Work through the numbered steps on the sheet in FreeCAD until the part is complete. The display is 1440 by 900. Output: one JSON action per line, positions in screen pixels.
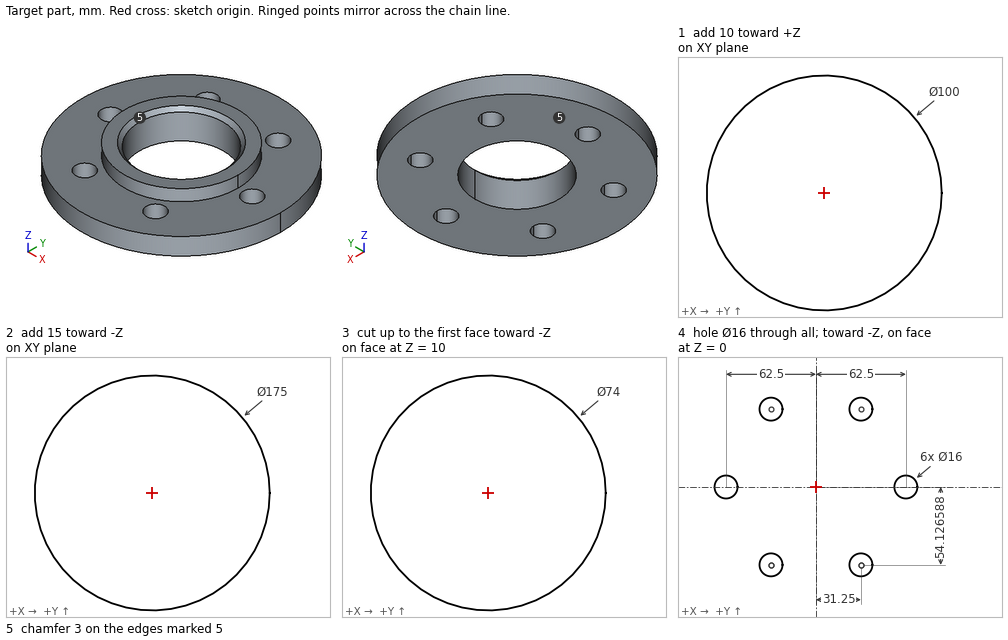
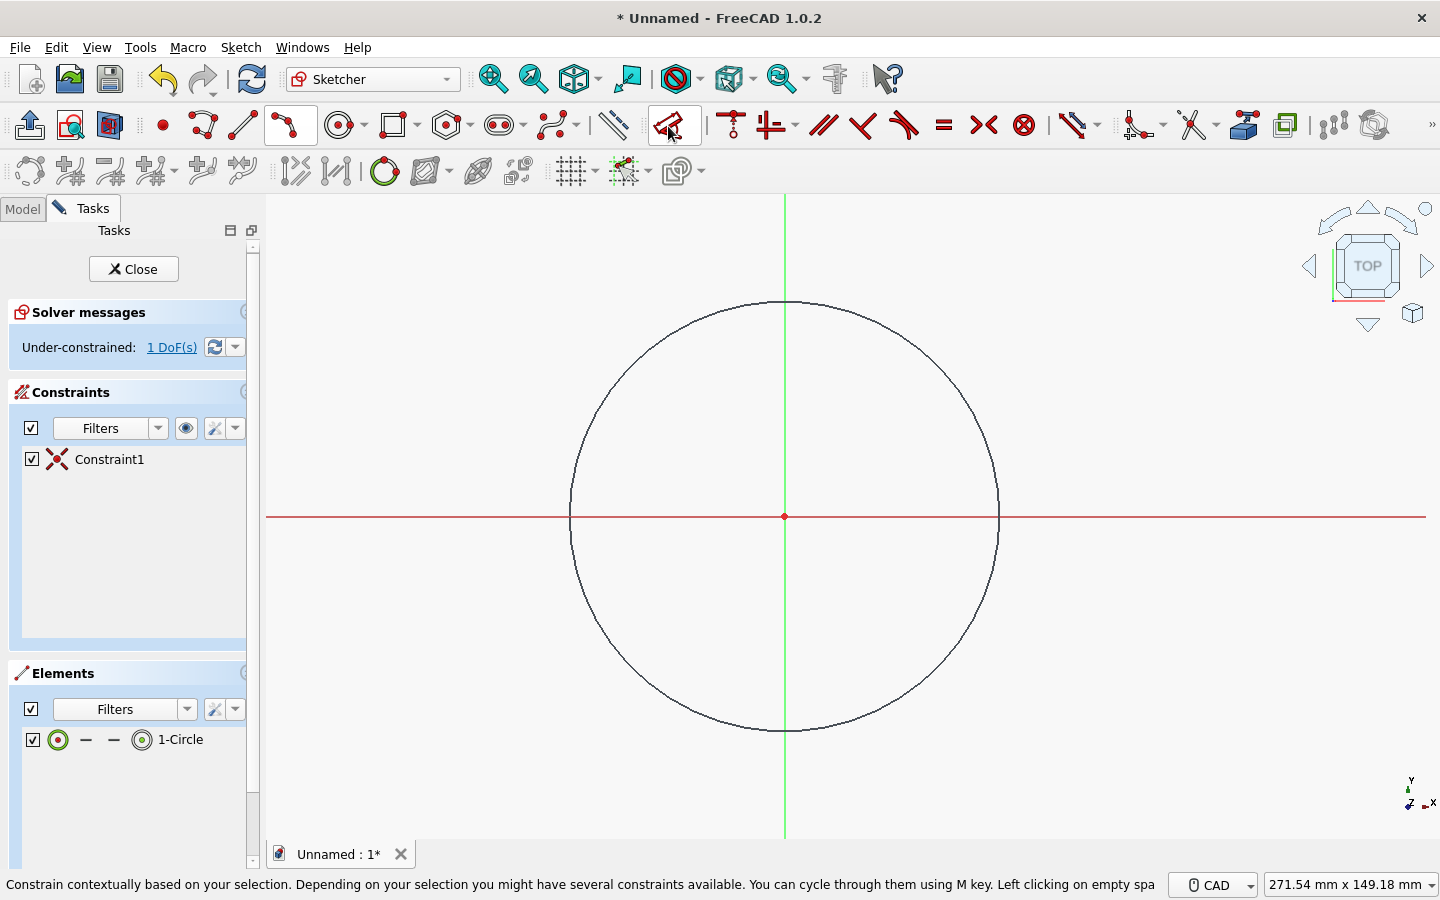
{"action": "left_click", "coordinate": [936, 364]}
{"action": "left_click", "coordinate": [959, 341]}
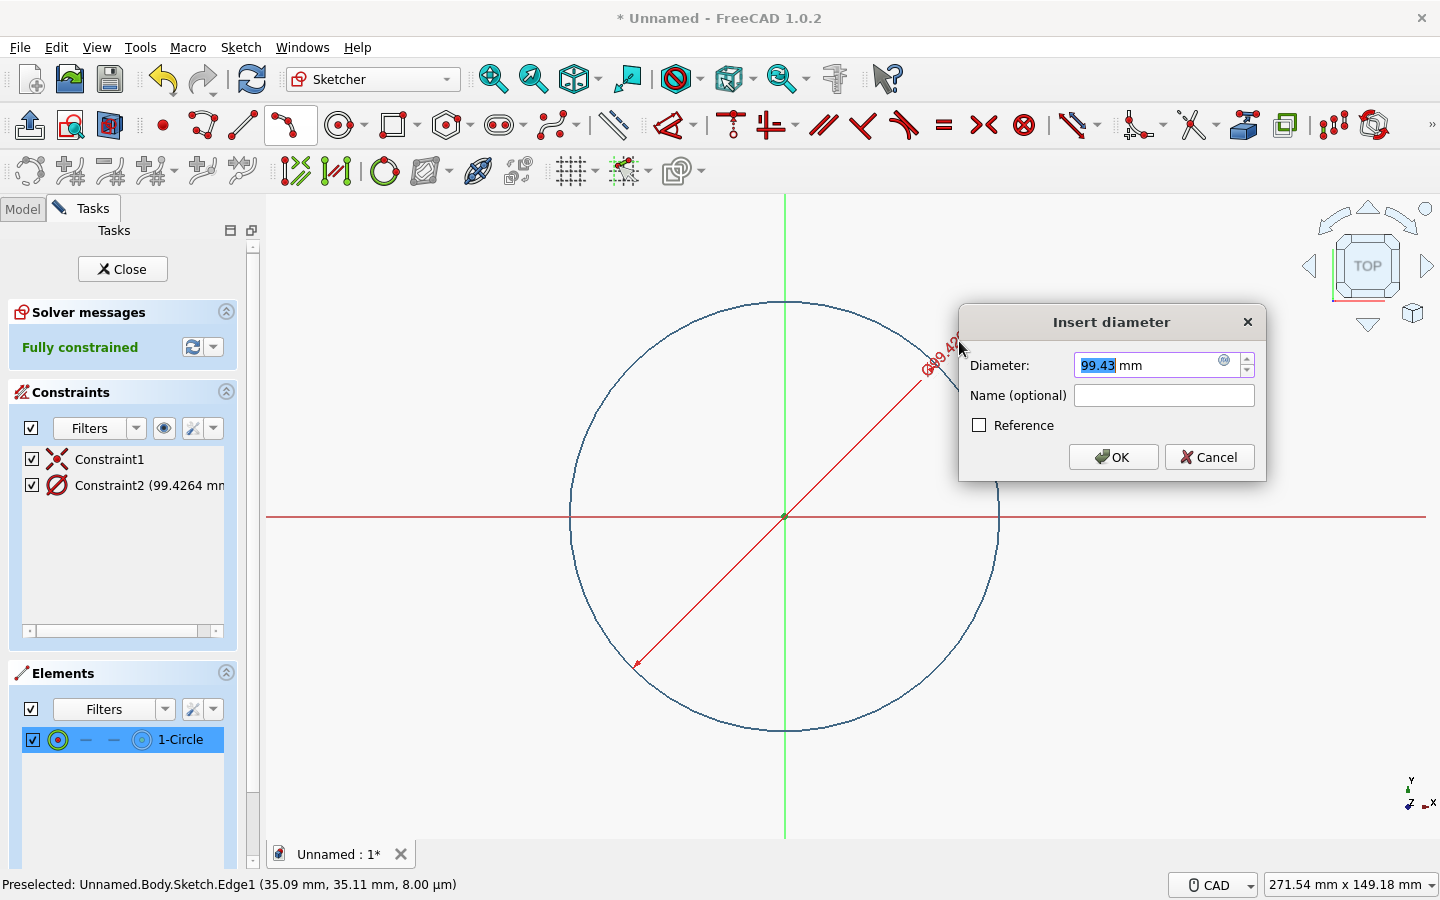
{"action": "type", "text": "100"}
{"action": "key", "text": "Return"}
{"action": "key", "text": "Escape"}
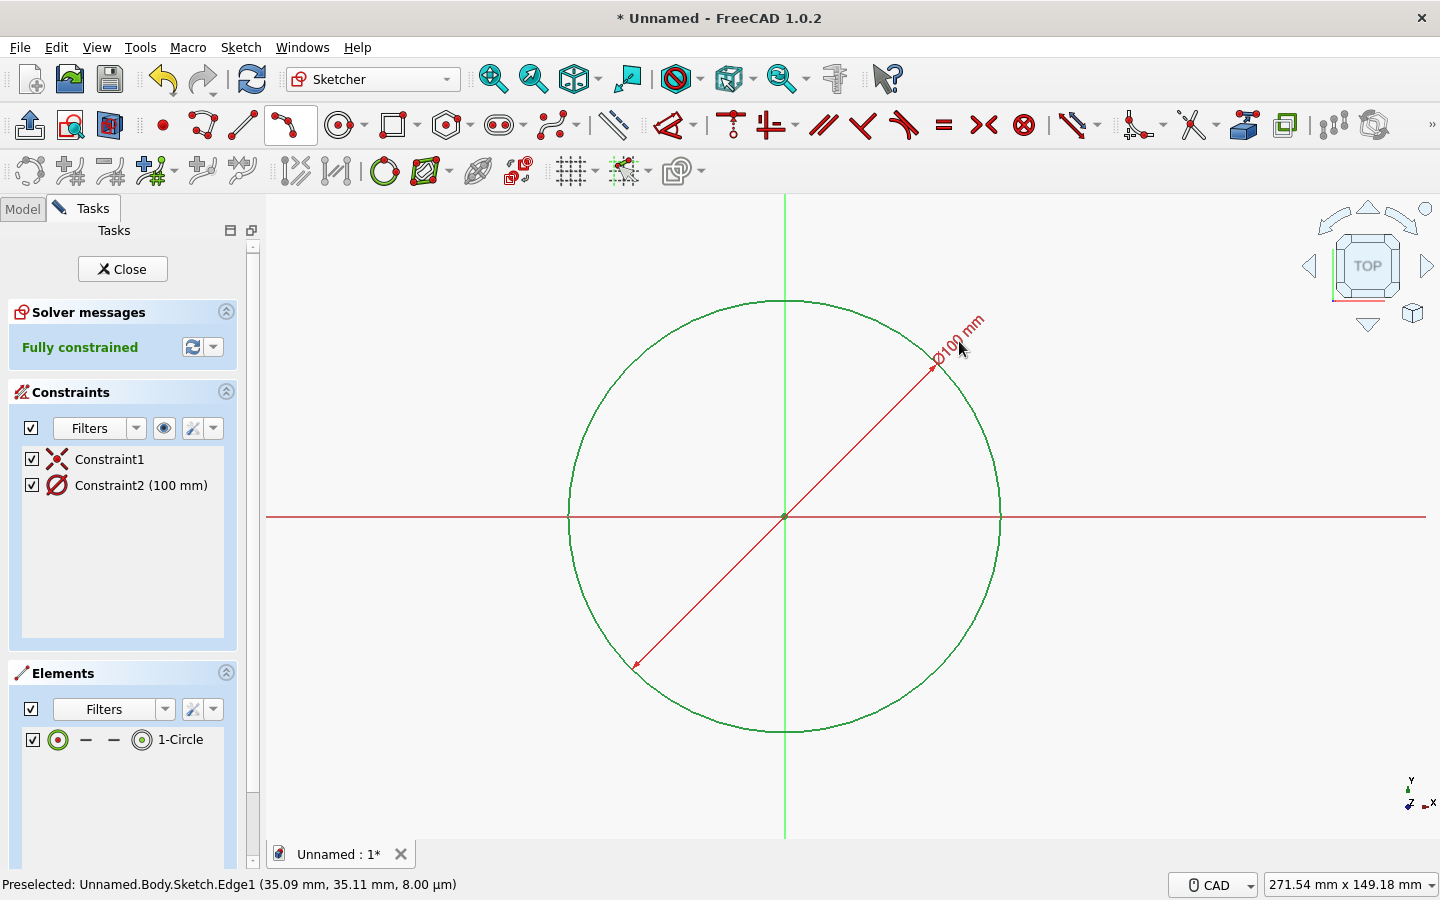
{"action": "left_click", "coordinate": [123, 269]}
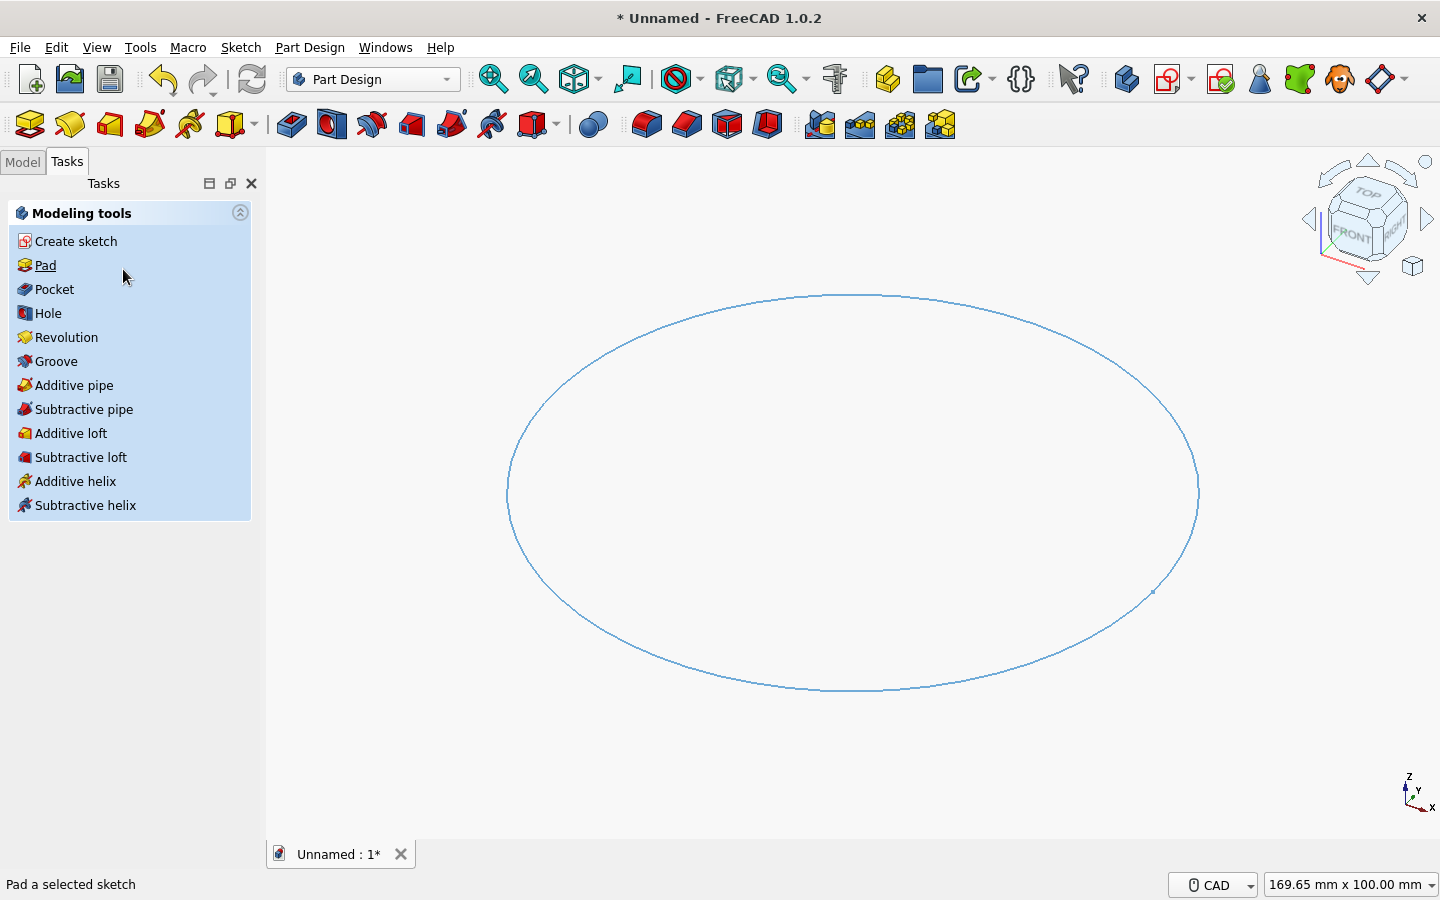
{"action": "left_click", "coordinate": [30, 124]}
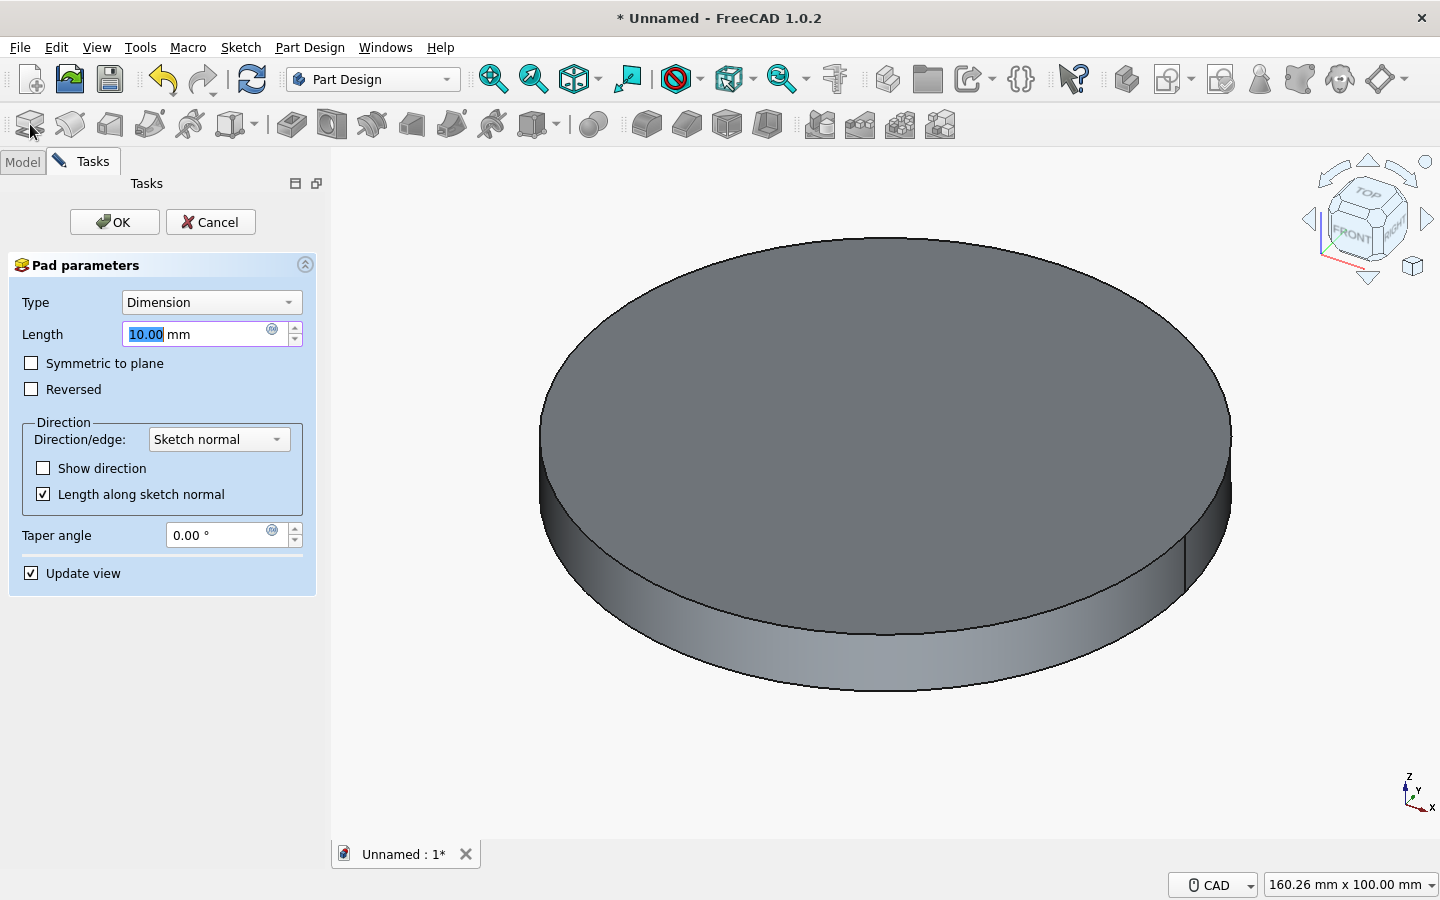
{"action": "type", "text": "10"}
{"action": "key", "text": "Tab"}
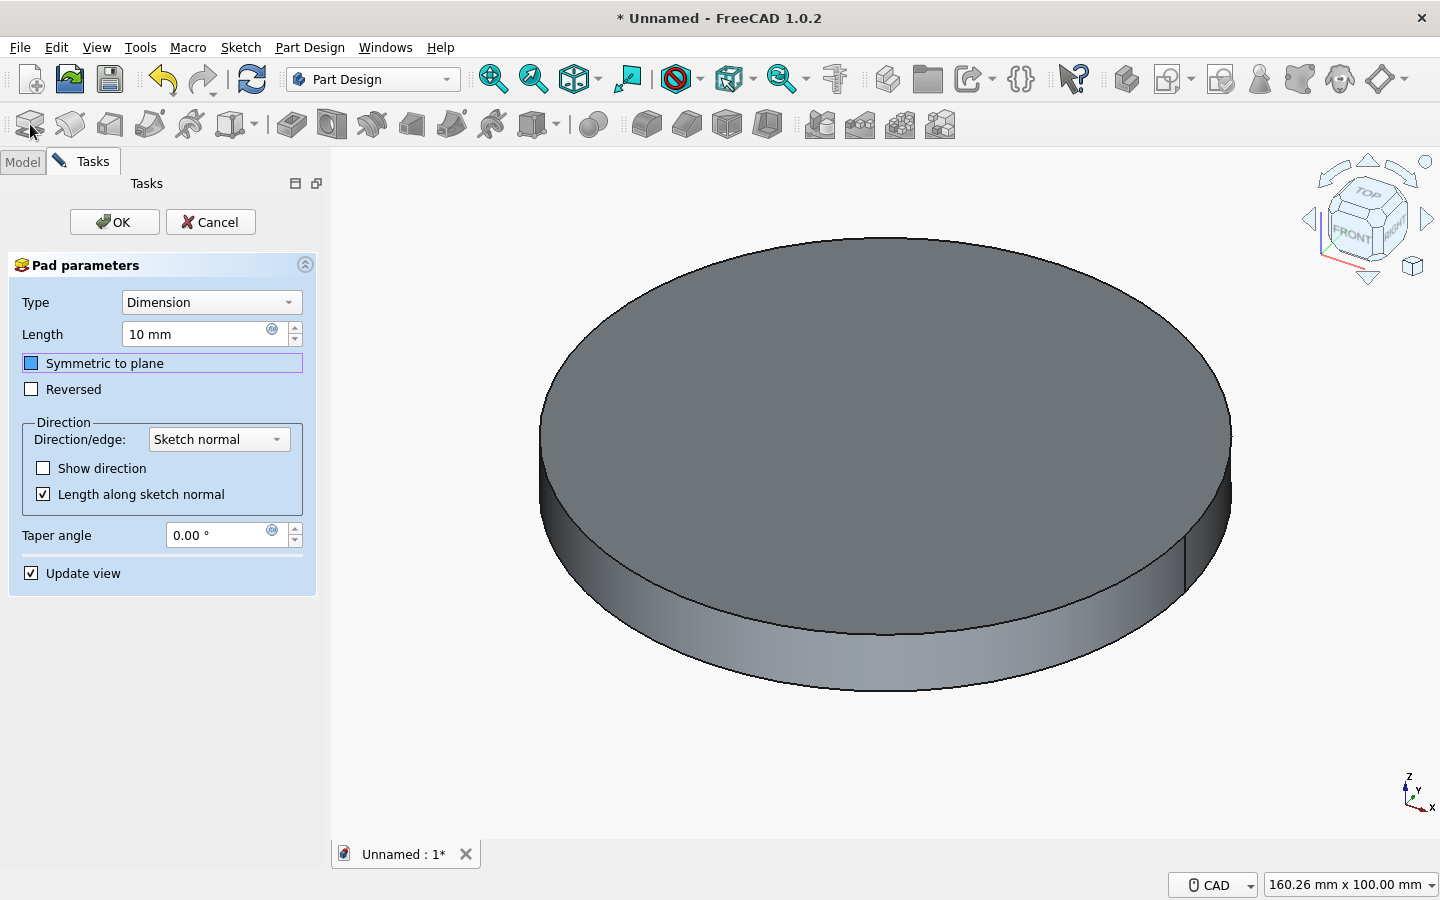
{"action": "left_click", "coordinate": [115, 222]}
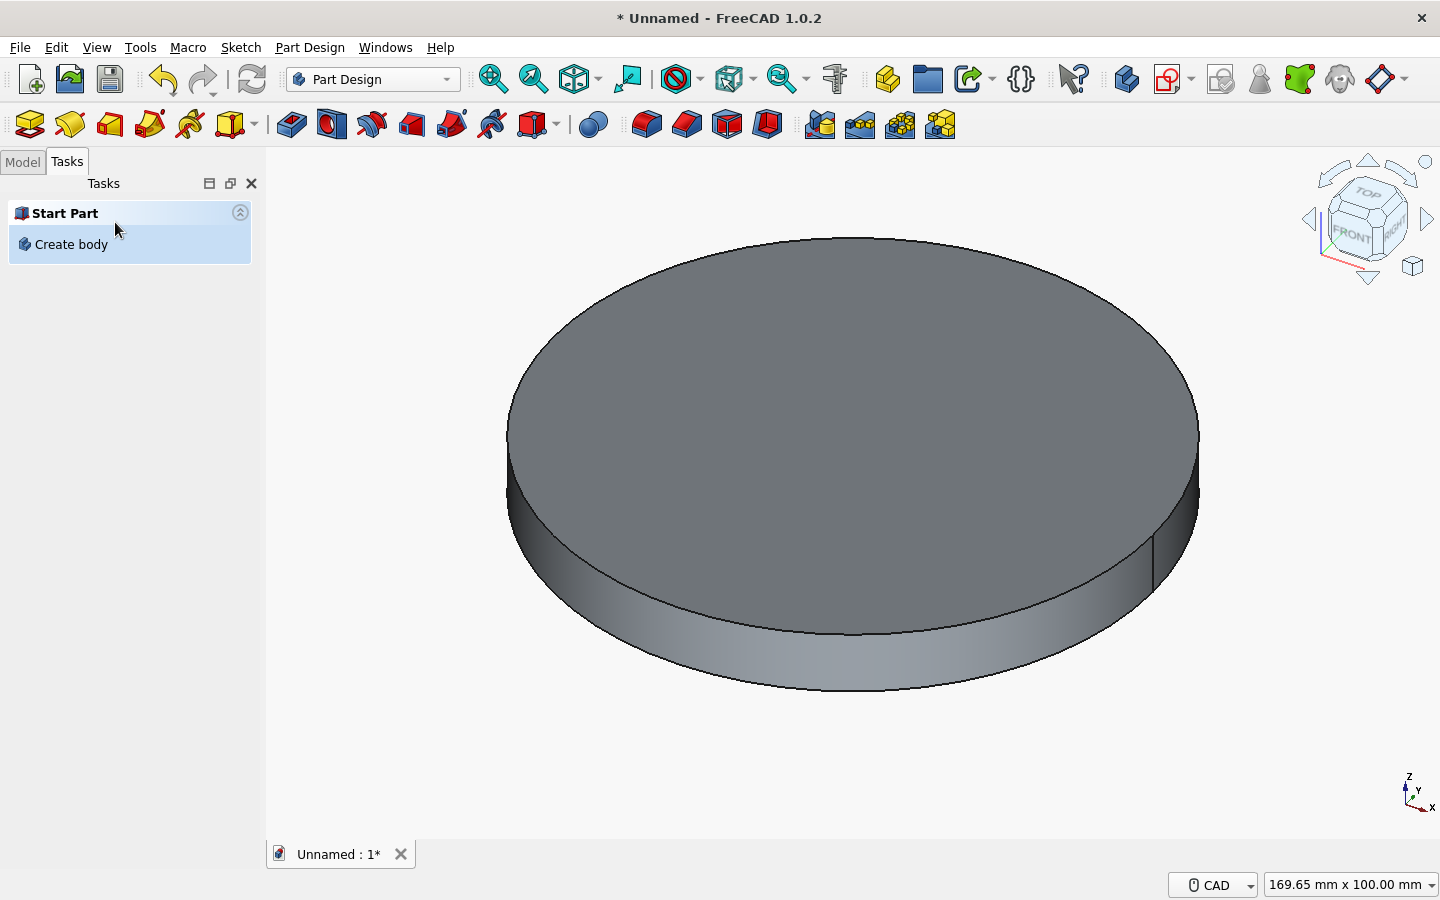
{"action": "left_click", "coordinate": [1168, 80]}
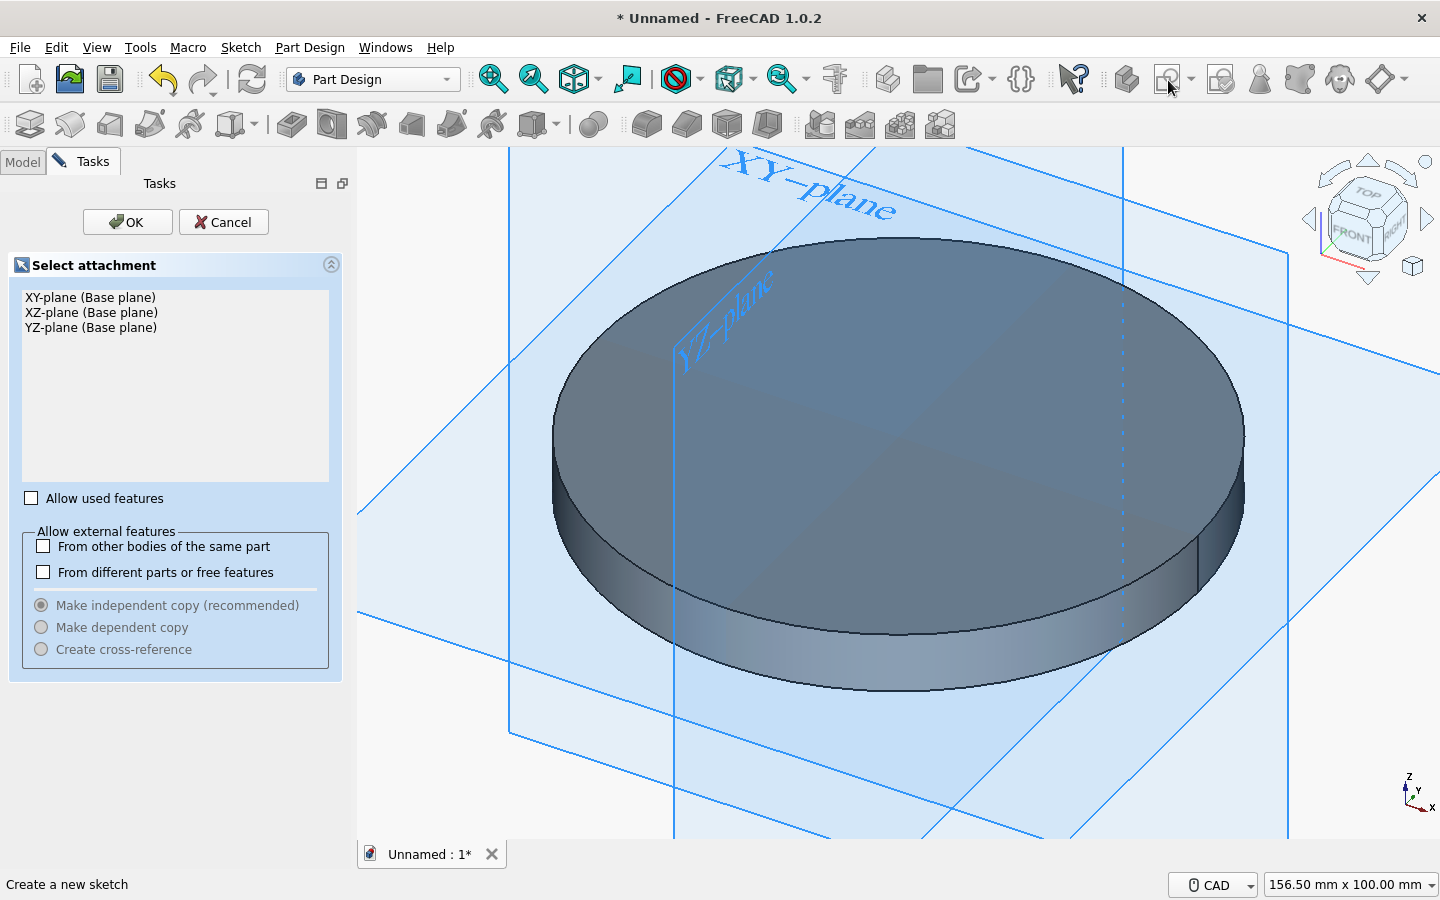
{"action": "left_click", "coordinate": [82, 298]}